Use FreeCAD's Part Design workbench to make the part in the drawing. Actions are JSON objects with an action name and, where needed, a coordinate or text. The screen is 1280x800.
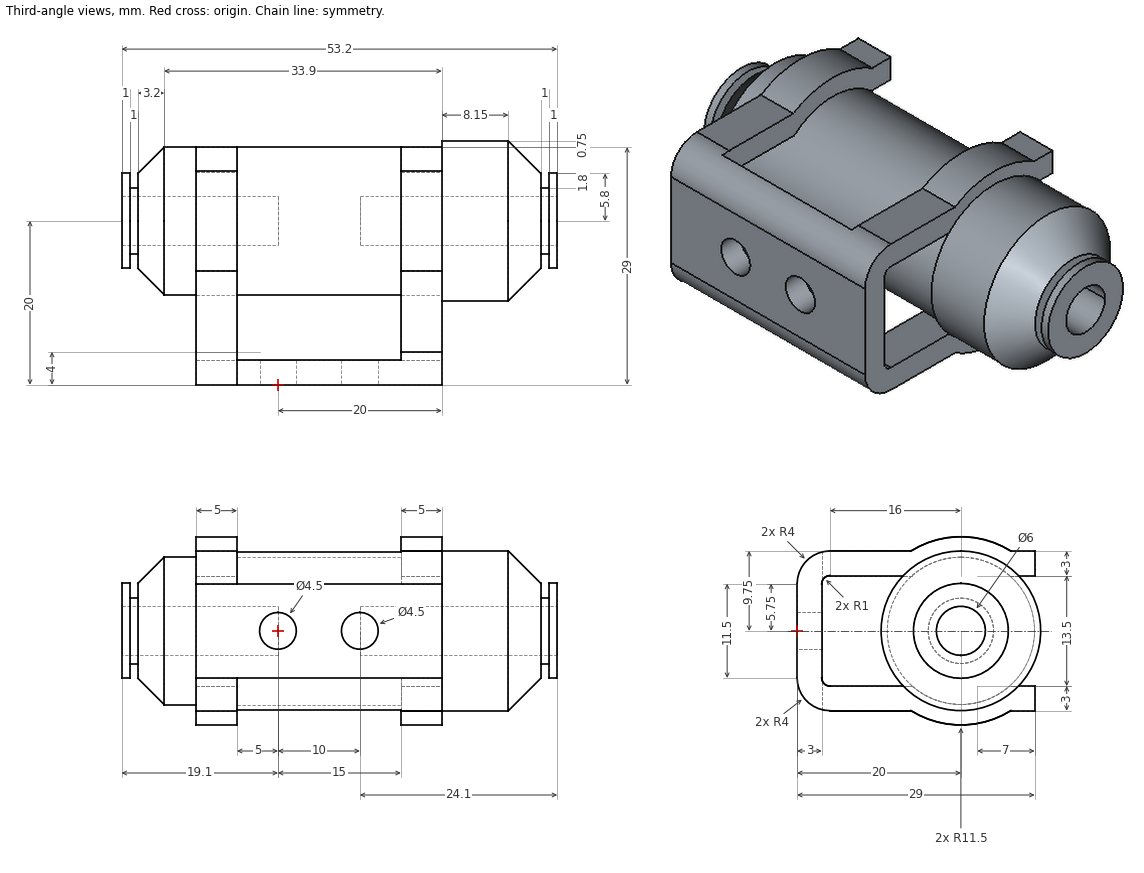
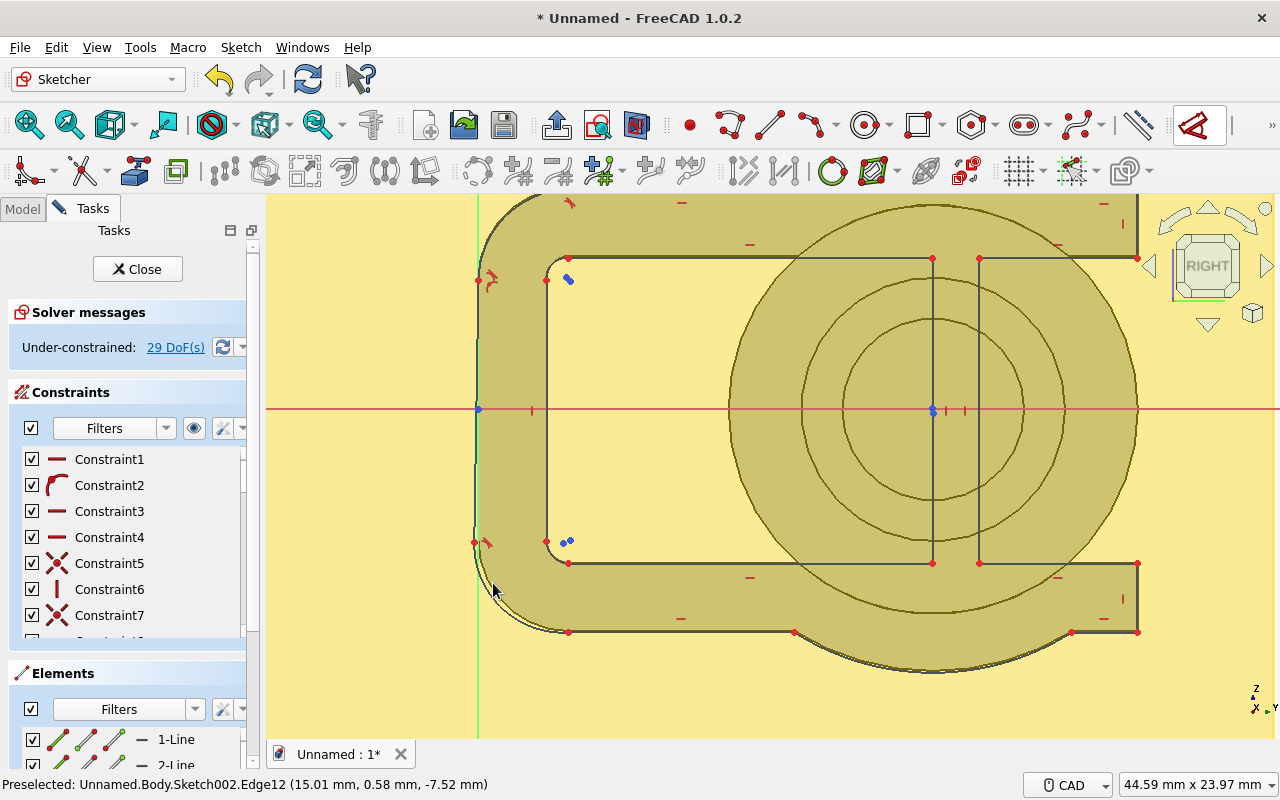
{"action": "left_click", "coordinate": [637, 632]}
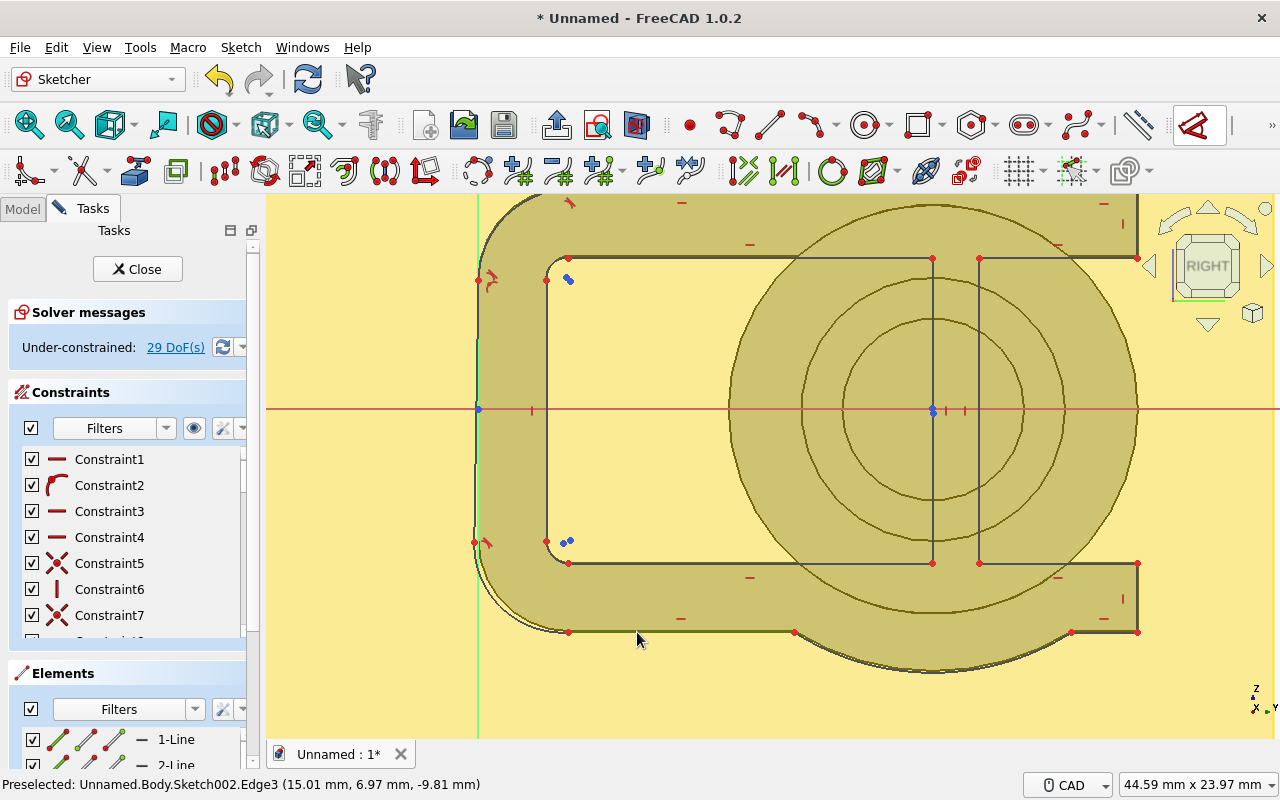
{"action": "left_click", "coordinate": [526, 625]}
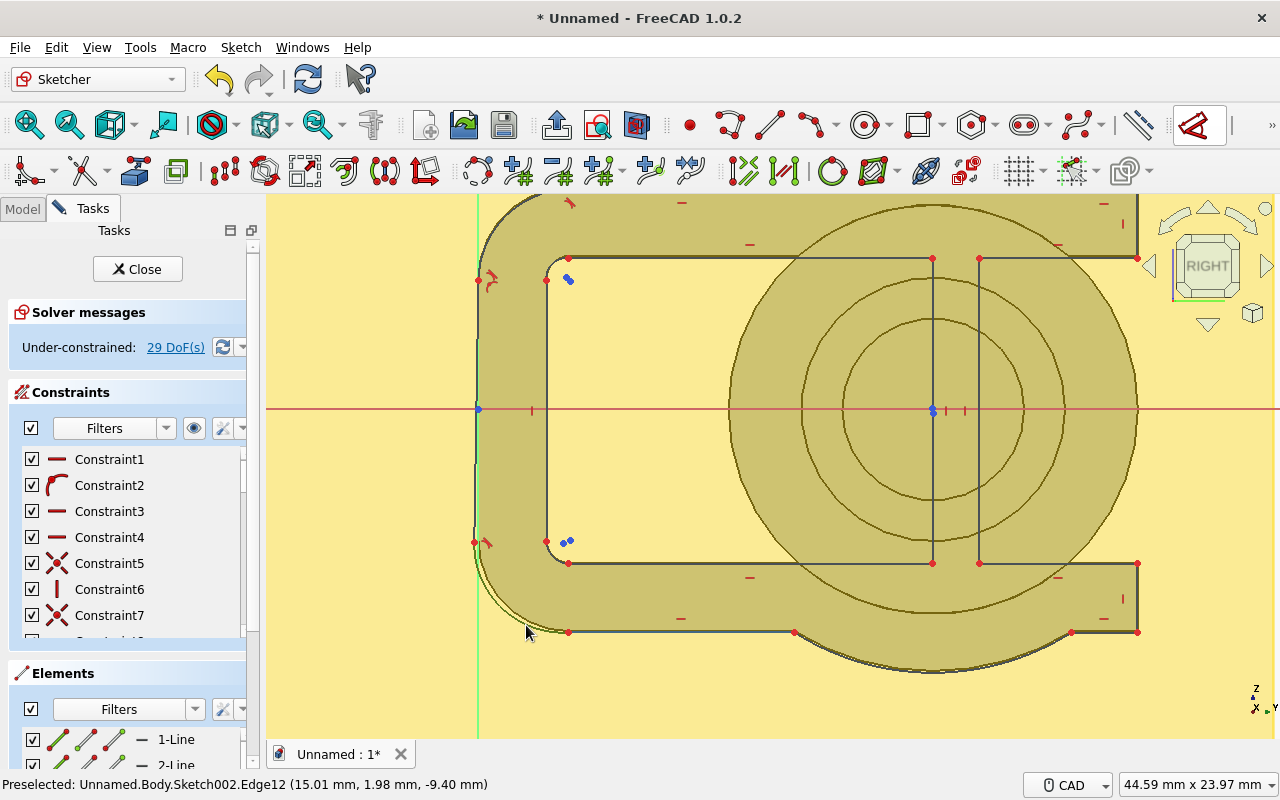
{"action": "key", "text": "t"}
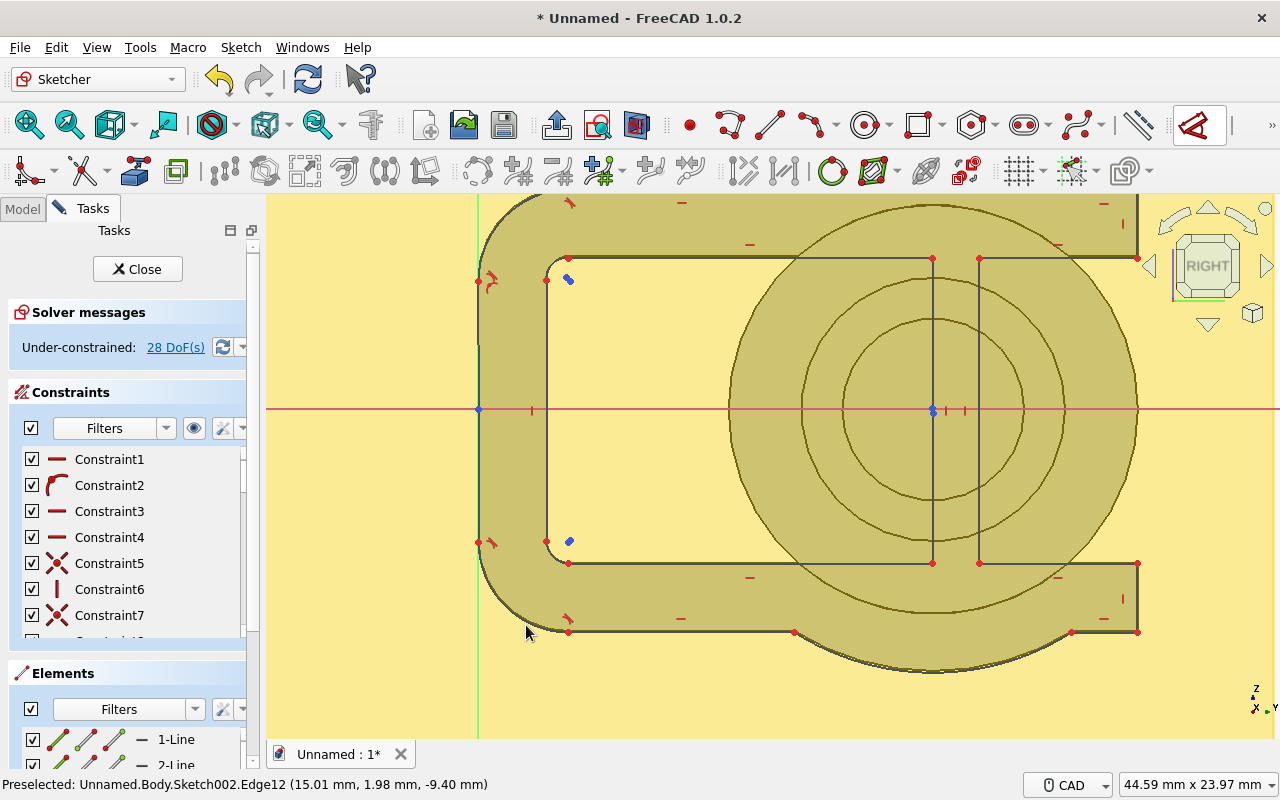
{"action": "left_click", "coordinate": [547, 463]}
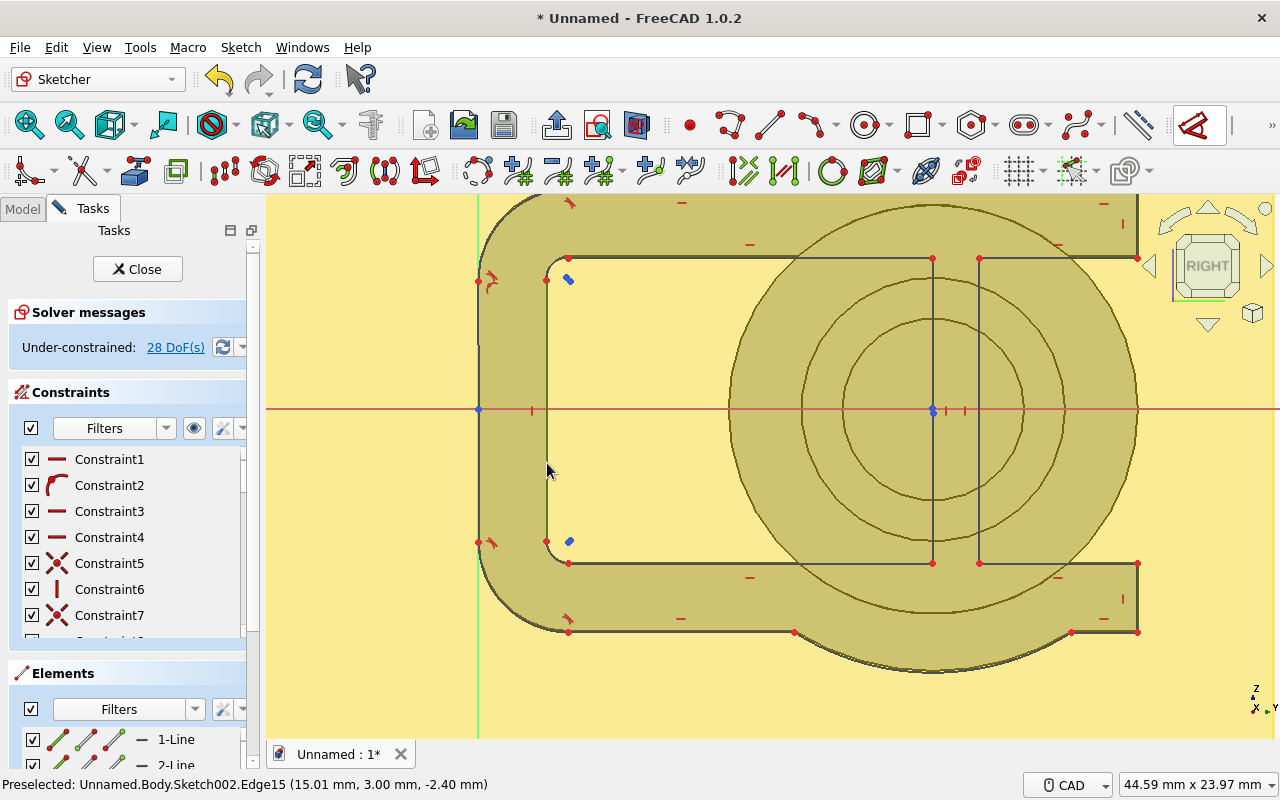
{"action": "scroll", "coordinate": [558, 260], "scroll_direction": "up", "scroll_amount": 2}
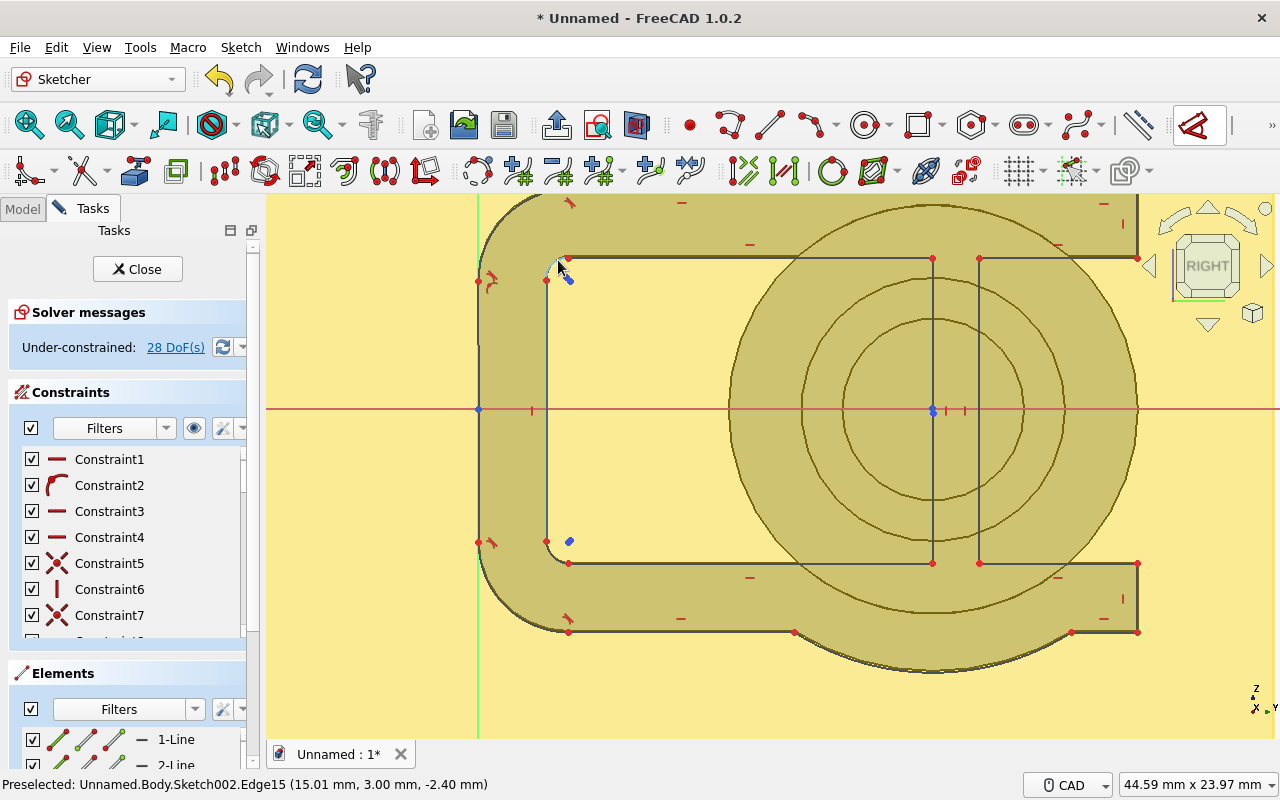
{"action": "left_click", "coordinate": [558, 259]}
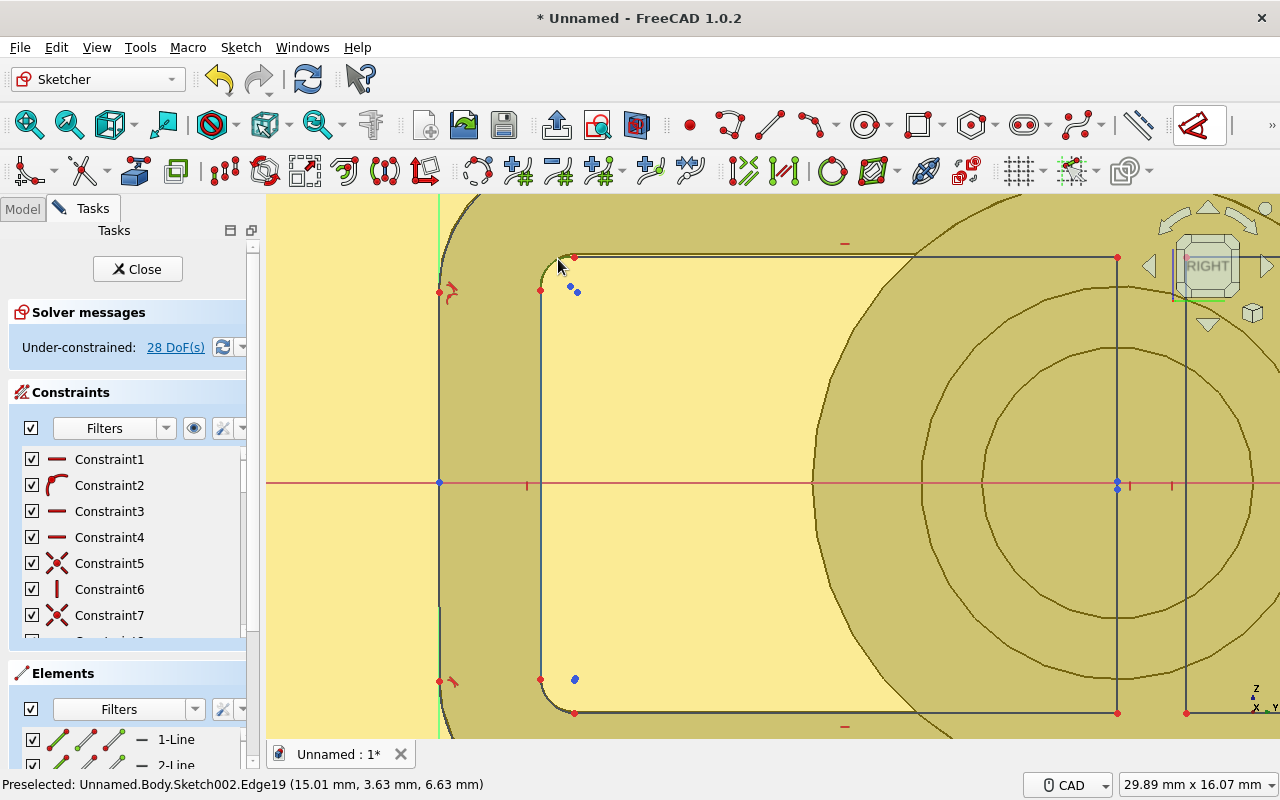
{"action": "key", "text": "t"}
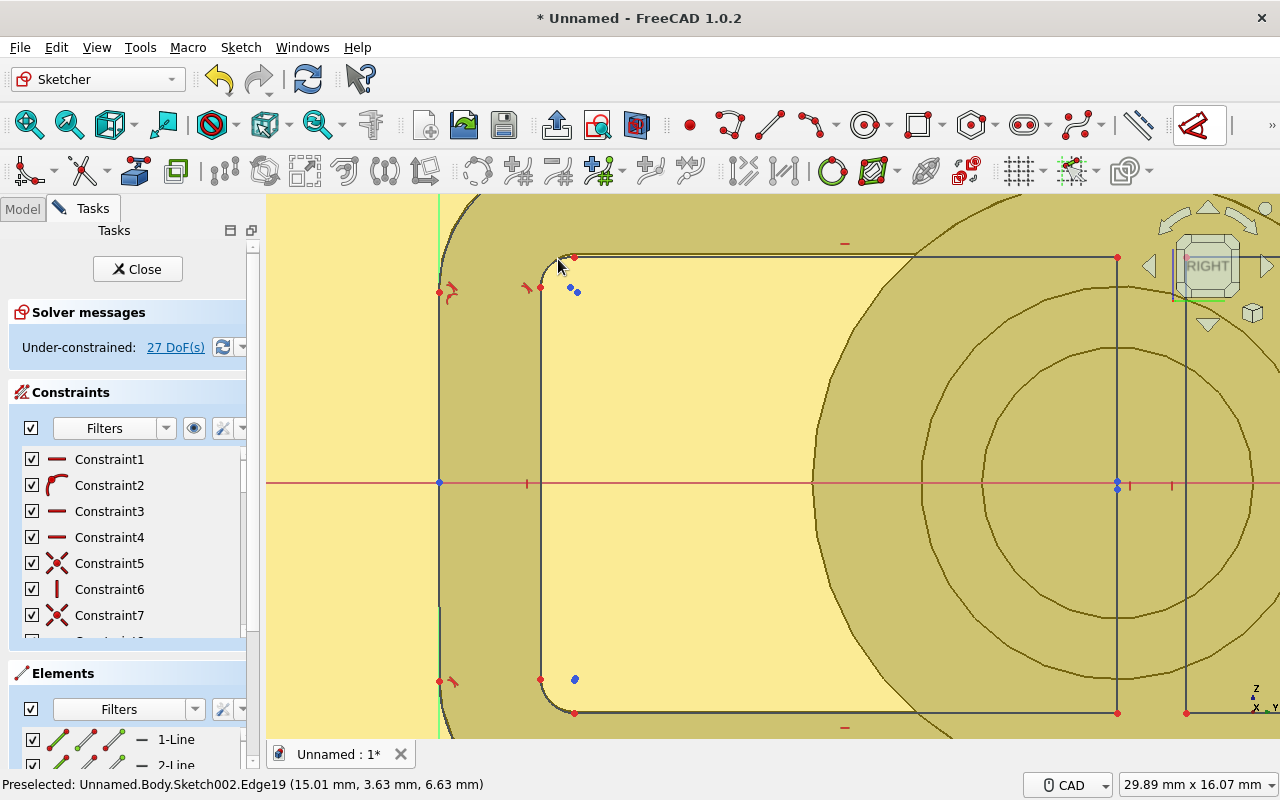
{"action": "left_click", "coordinate": [541, 562]}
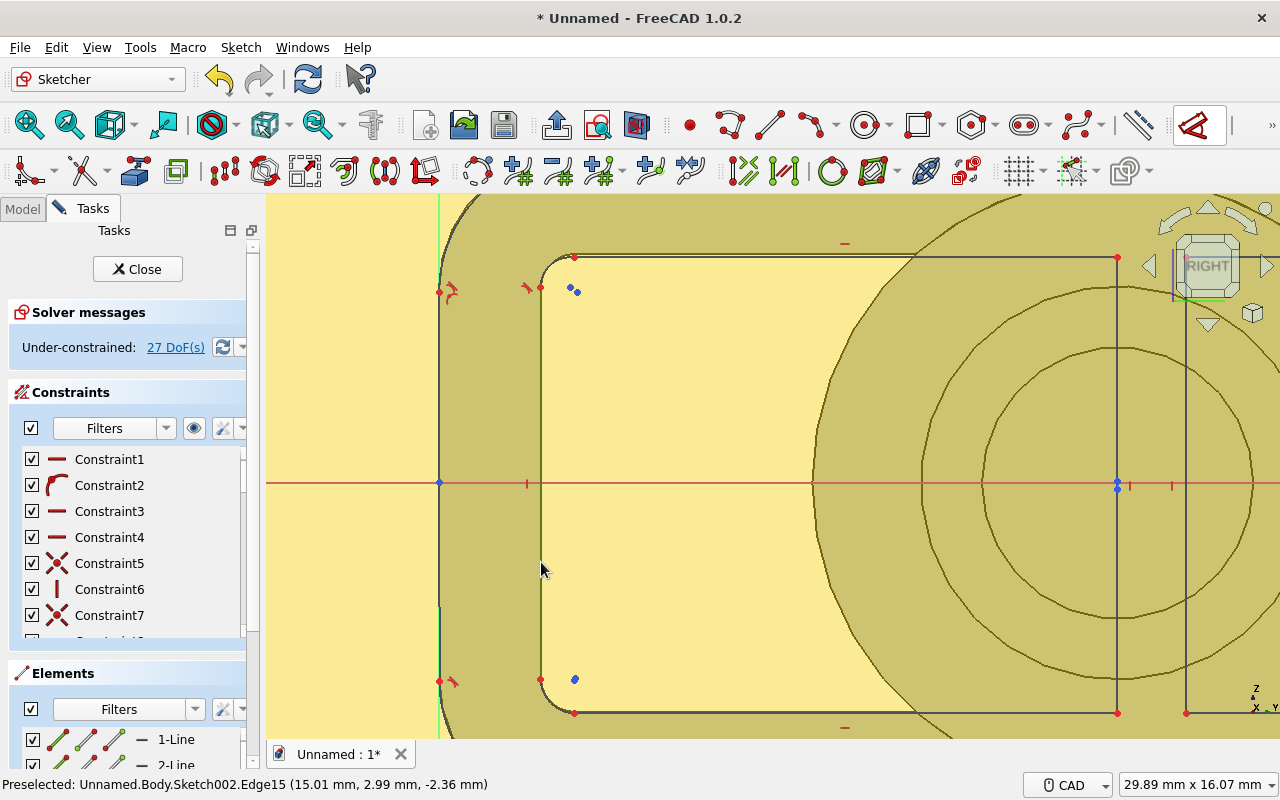
{"action": "left_click", "coordinate": [545, 695]}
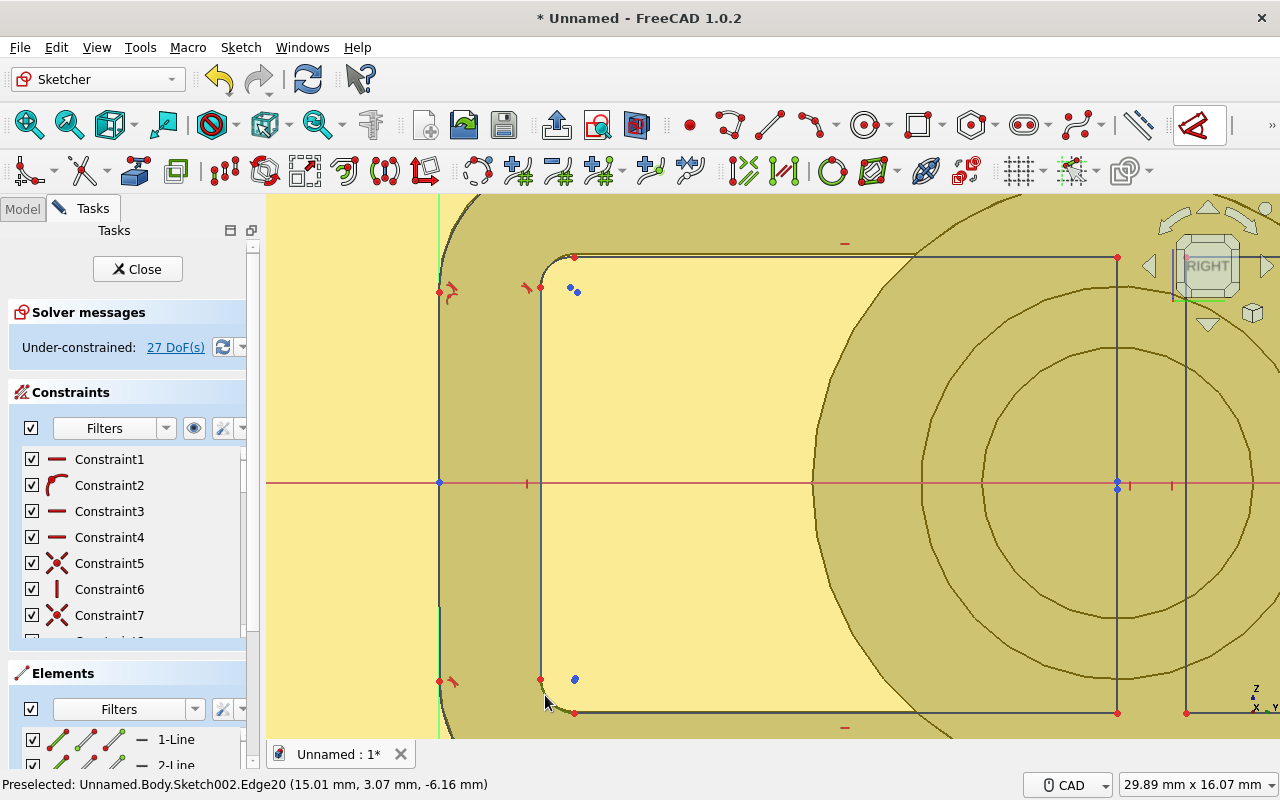
{"action": "key", "text": "t"}